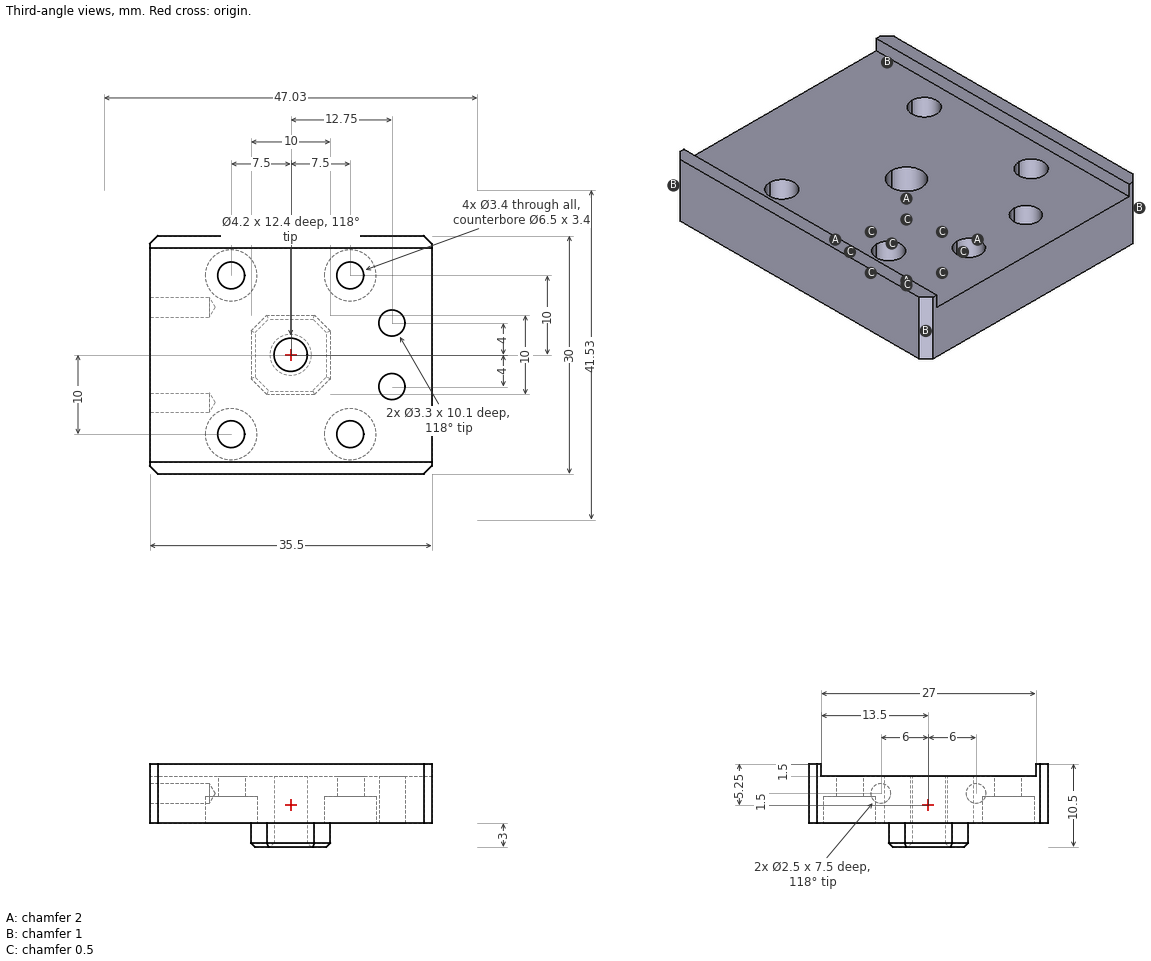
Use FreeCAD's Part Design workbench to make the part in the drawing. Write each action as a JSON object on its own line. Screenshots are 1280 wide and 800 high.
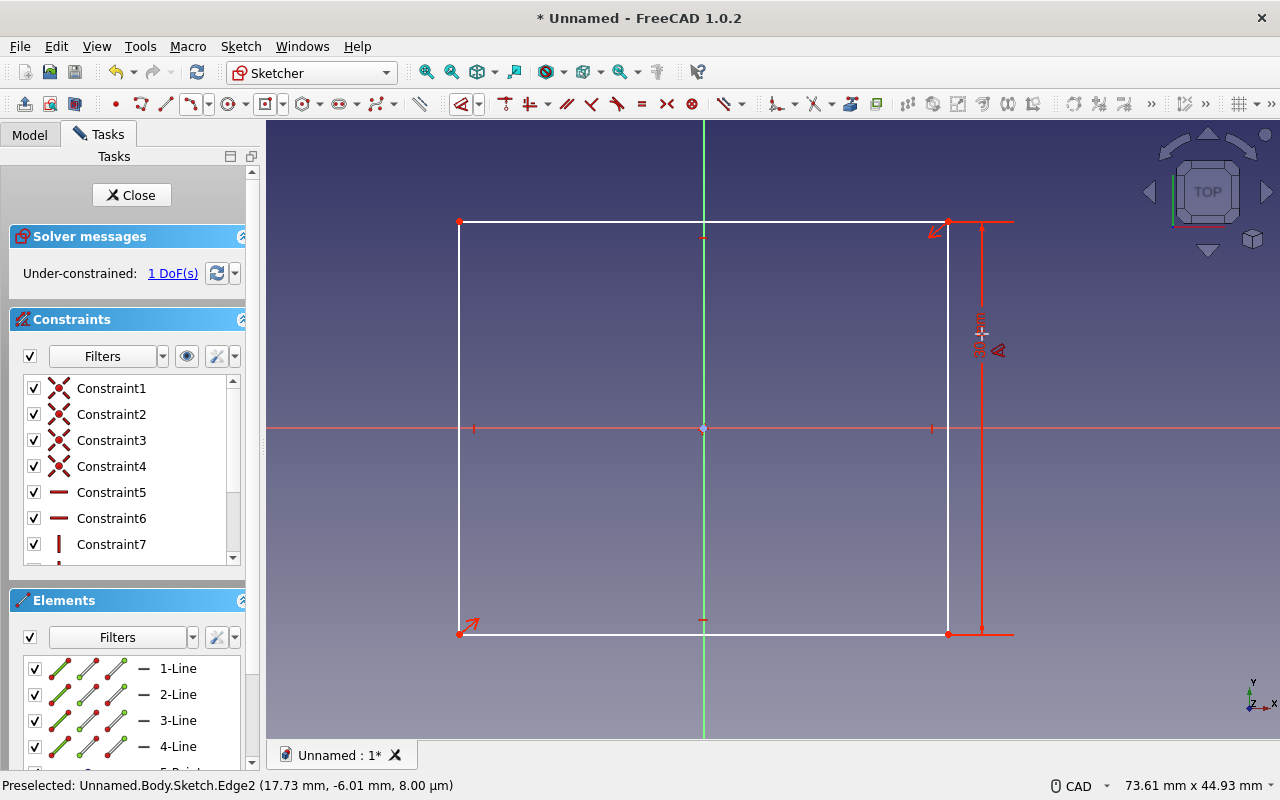
{"action": "left_click", "coordinate": [606, 635]}
{"action": "left_click", "coordinate": [591, 669]}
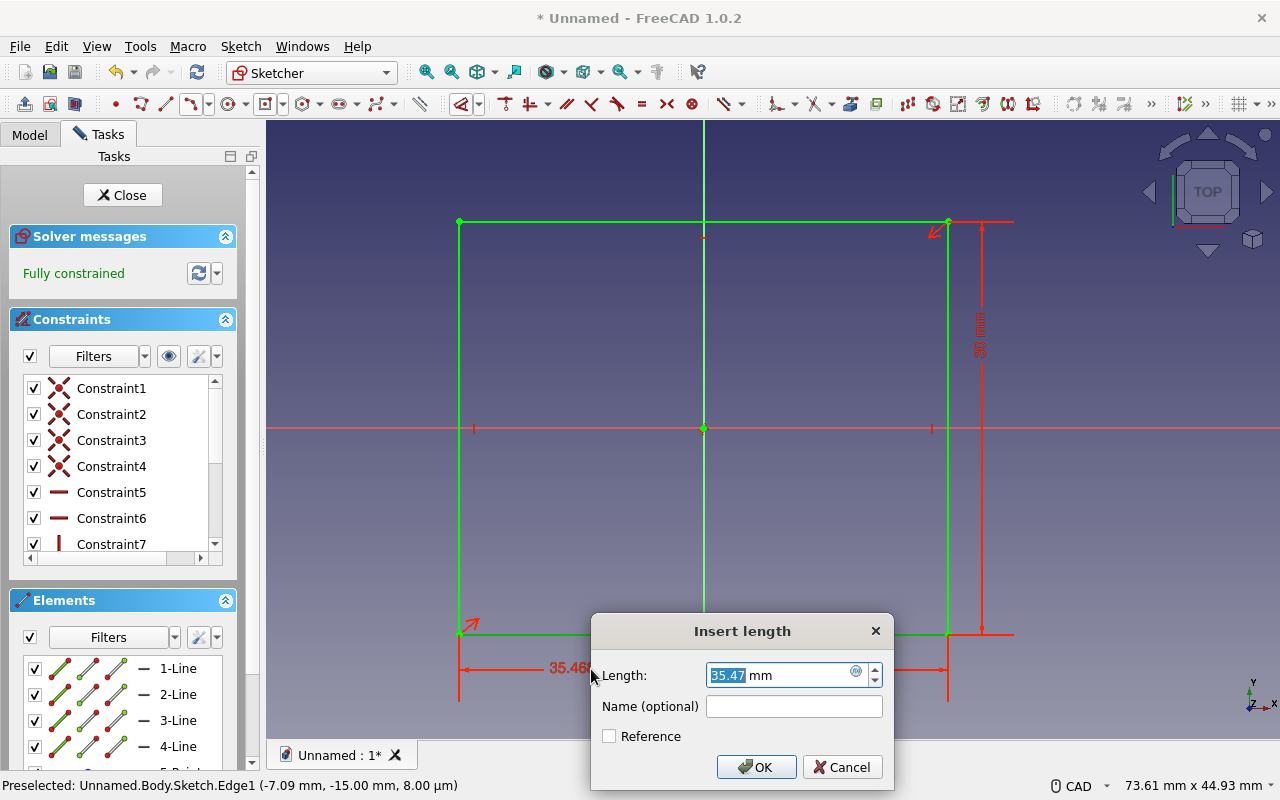
{"action": "type", "text": "35.5"}
{"action": "key", "text": "Return"}
{"action": "key", "text": "Escape"}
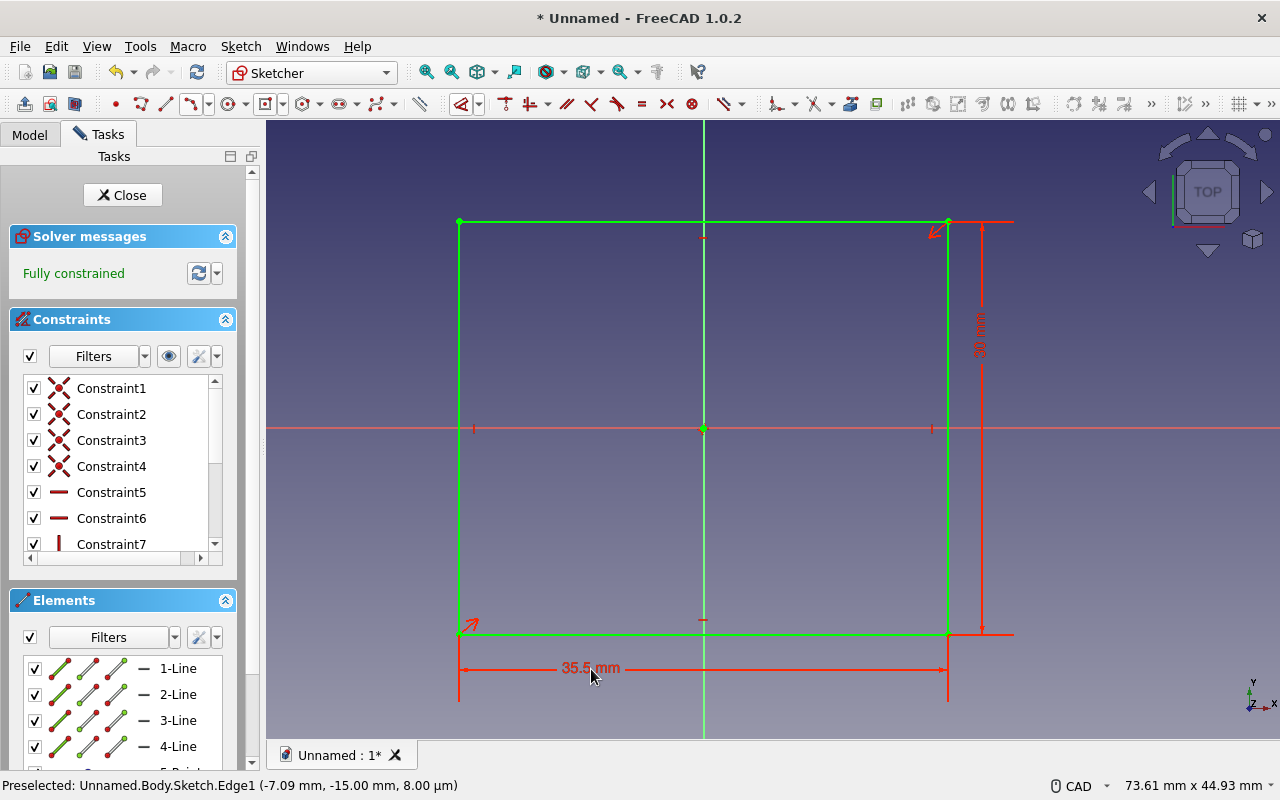
{"action": "left_click", "coordinate": [123, 195]}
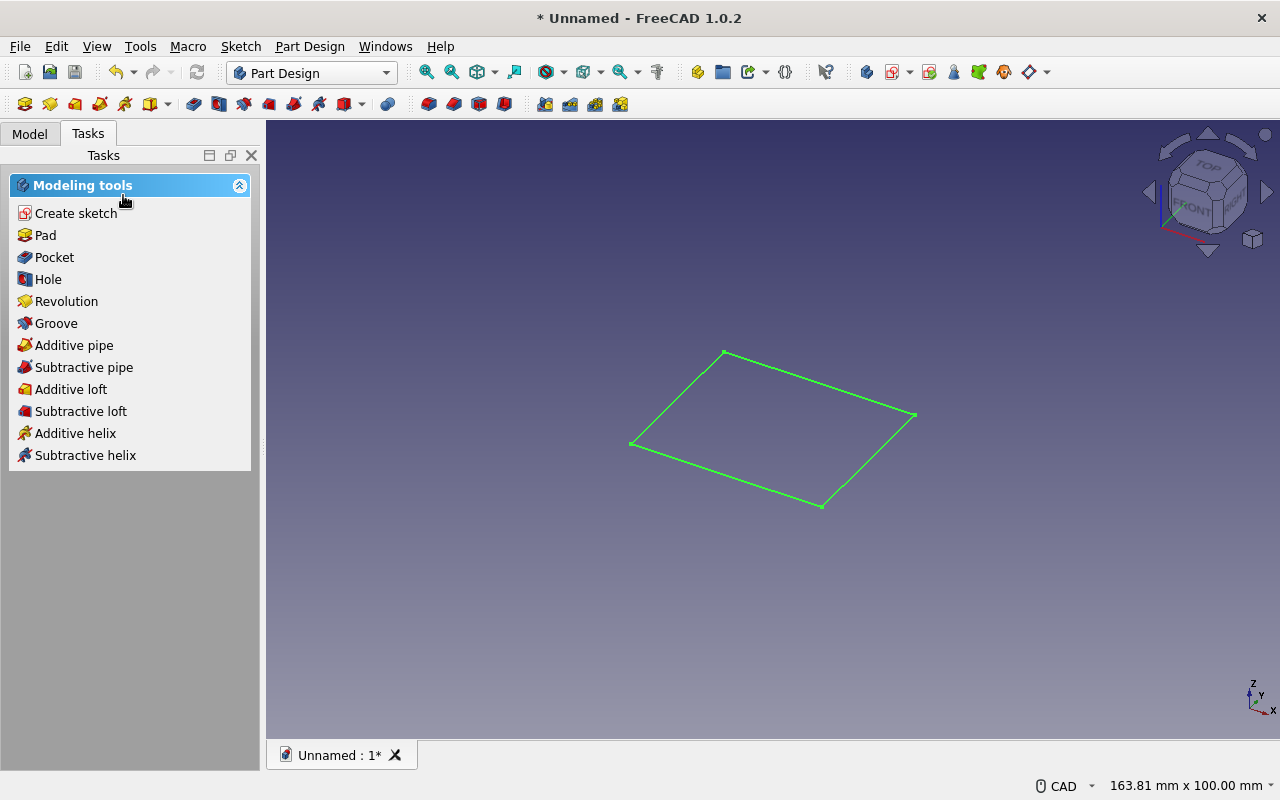
{"action": "left_click", "coordinate": [25, 104]}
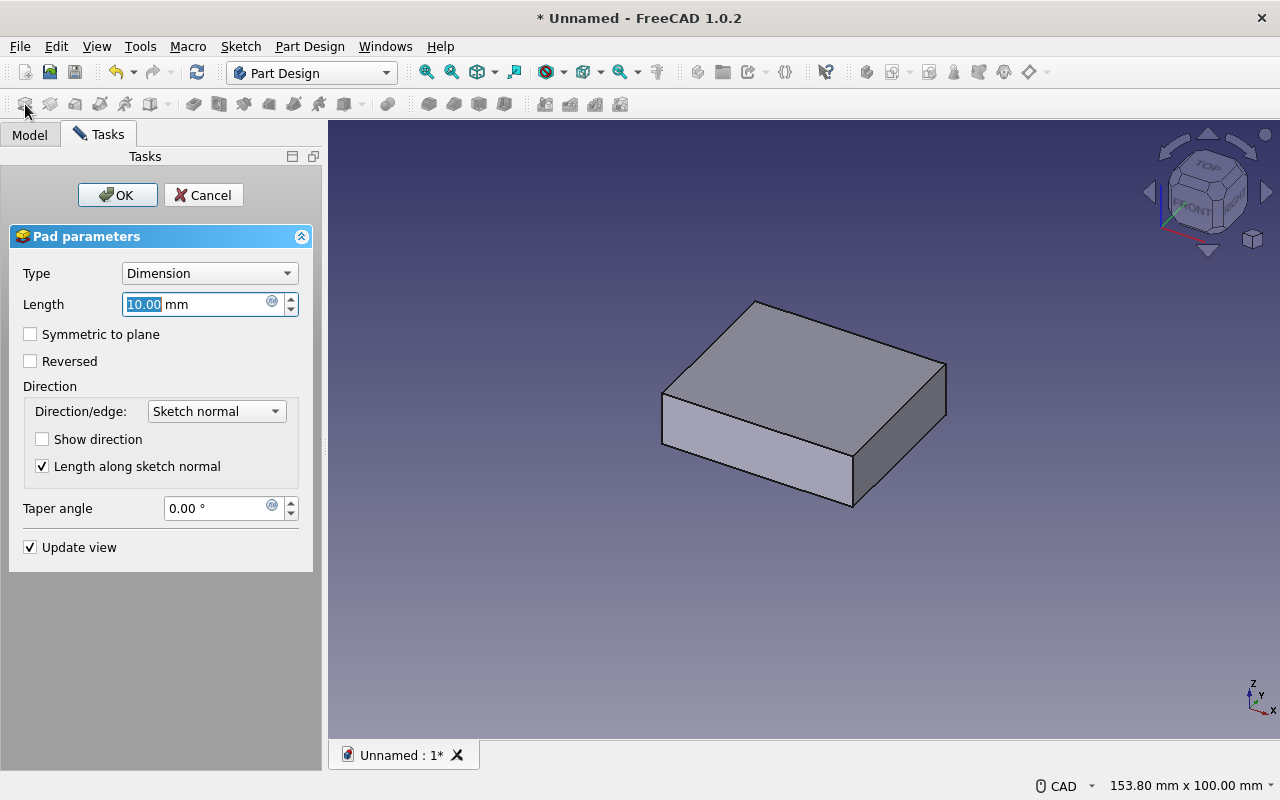
{"action": "type", "text": "10.5"}
{"action": "key", "text": "Tab"}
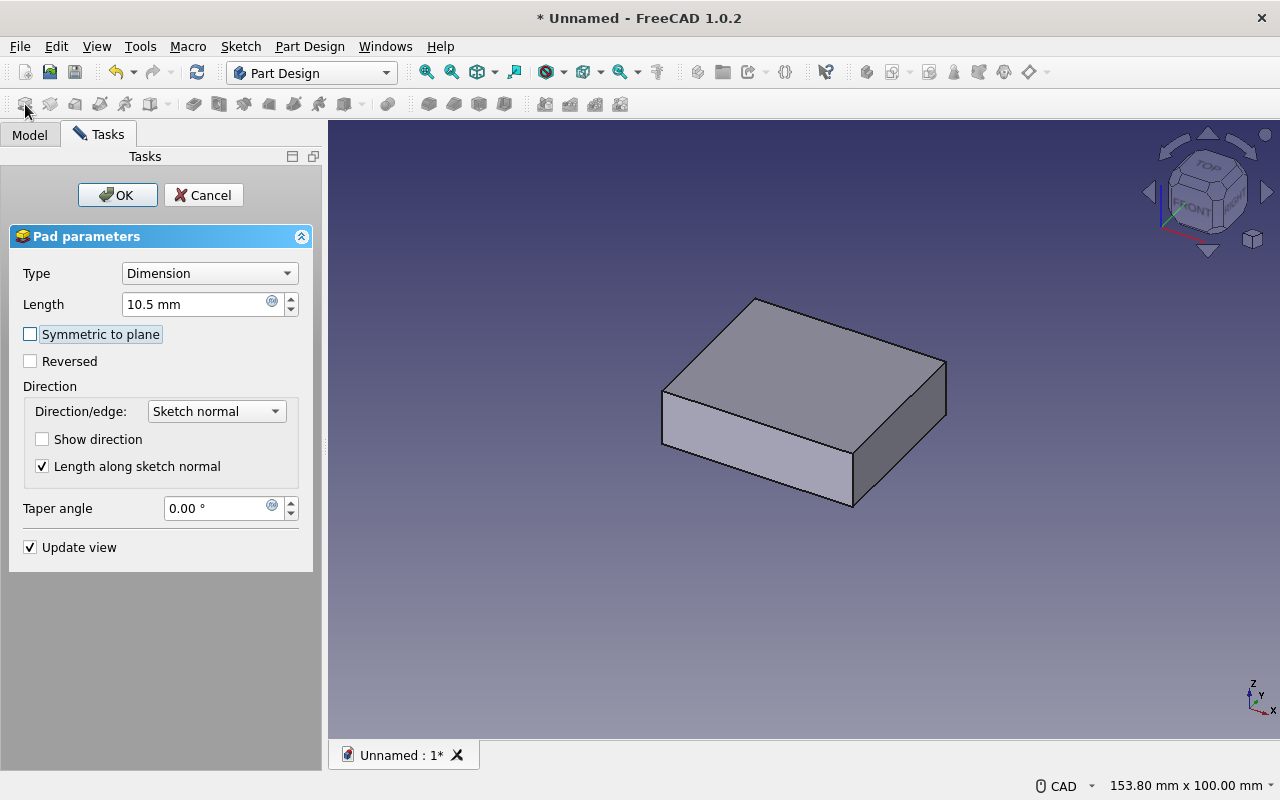
{"action": "left_click", "coordinate": [31, 334]}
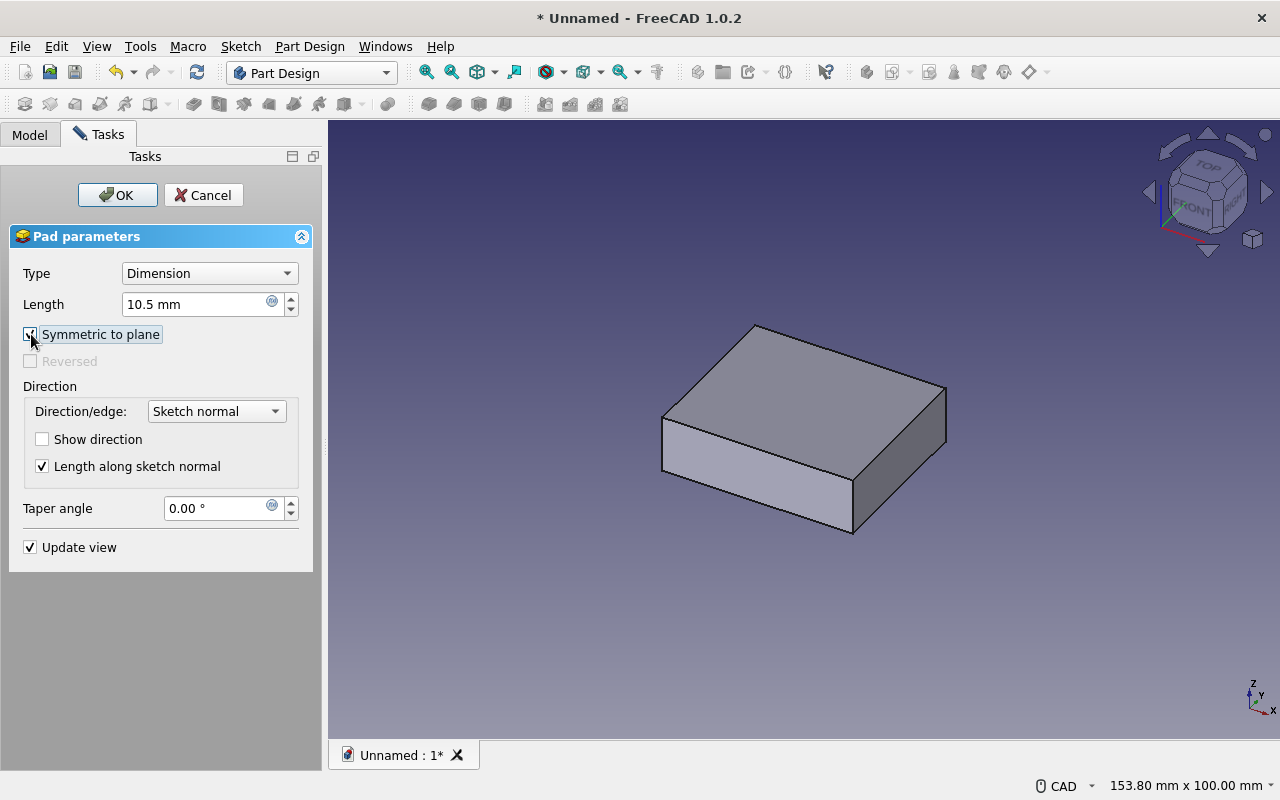
{"action": "left_click", "coordinate": [118, 195]}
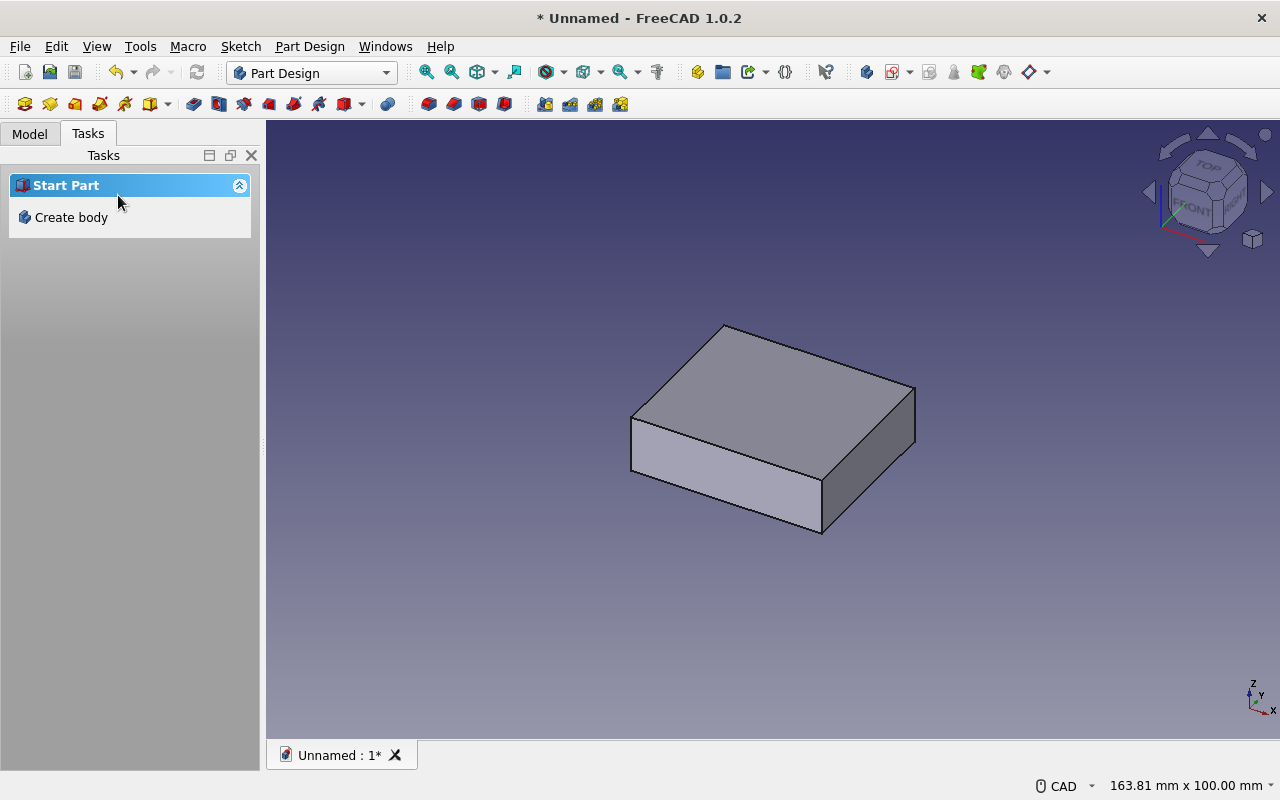
{"action": "left_click", "coordinate": [427, 72]}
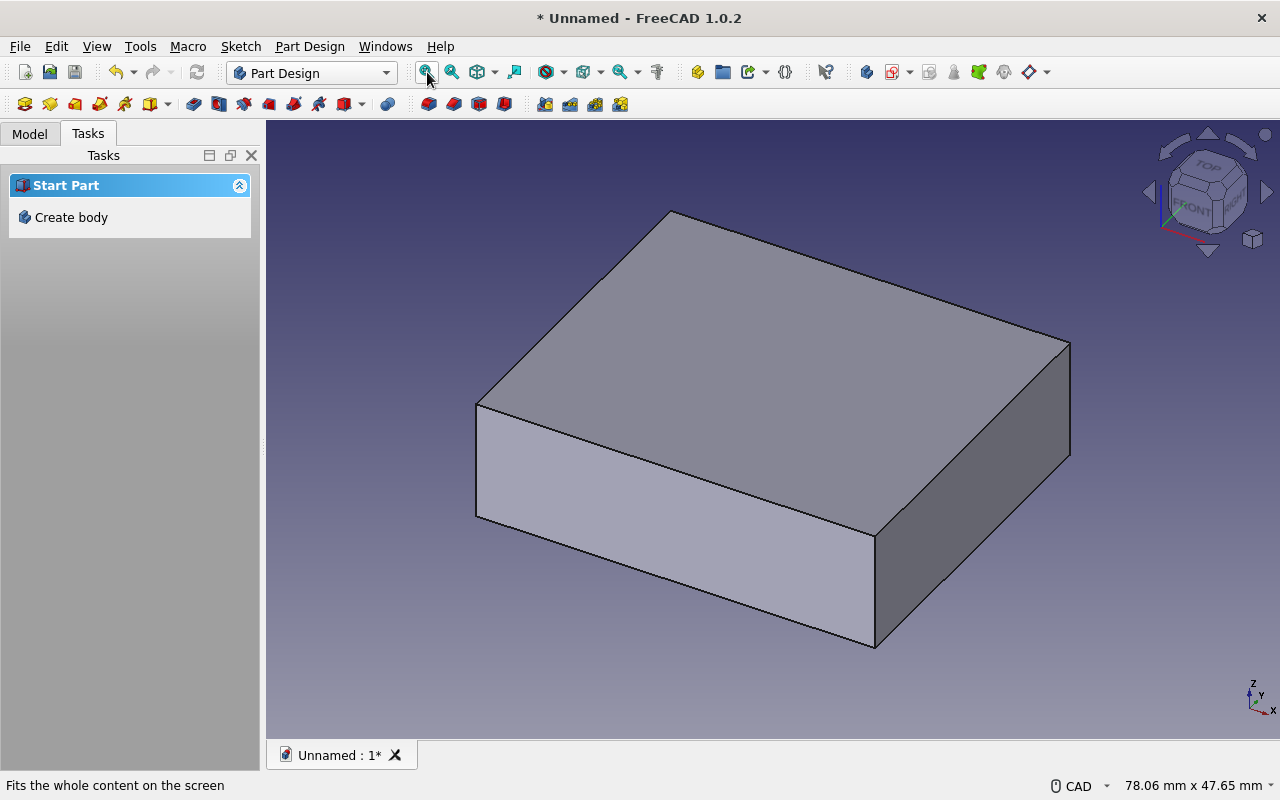
{"action": "left_click", "coordinate": [1028, 439]}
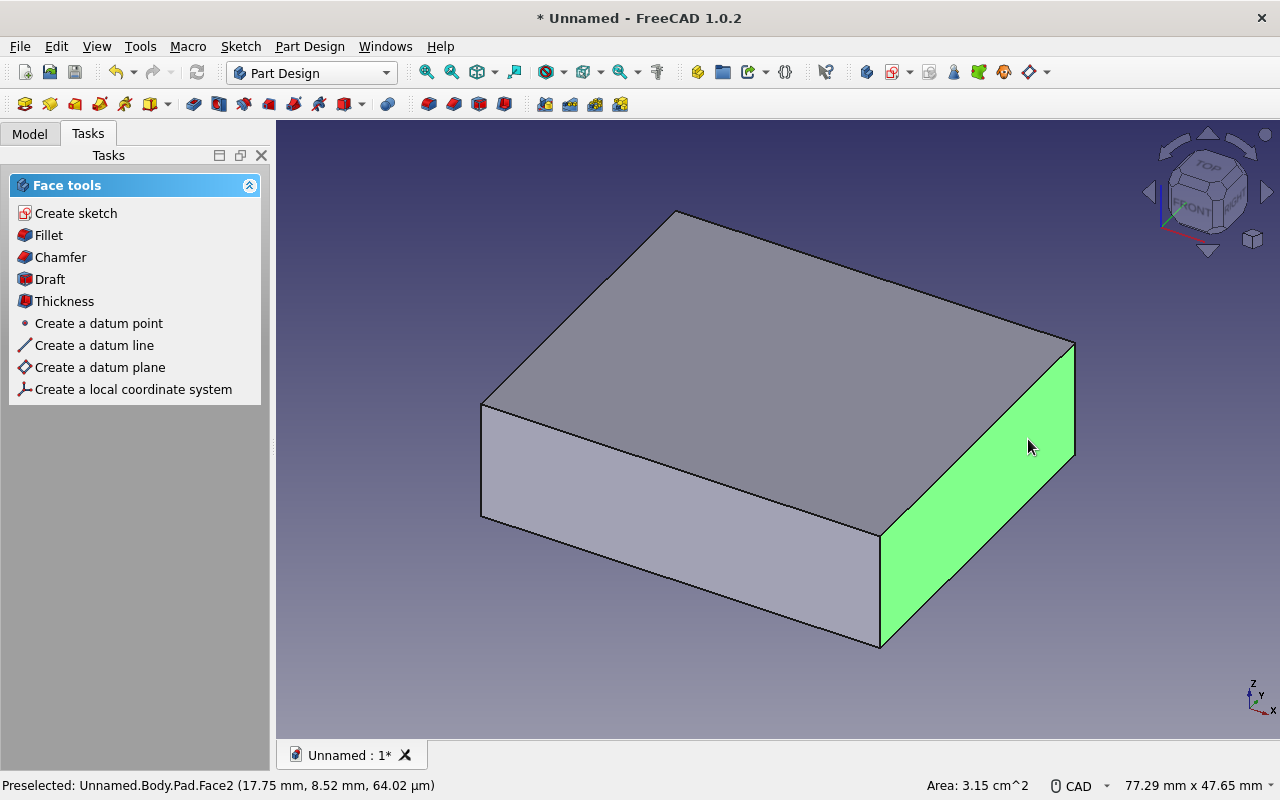
{"action": "left_click", "coordinate": [892, 72]}